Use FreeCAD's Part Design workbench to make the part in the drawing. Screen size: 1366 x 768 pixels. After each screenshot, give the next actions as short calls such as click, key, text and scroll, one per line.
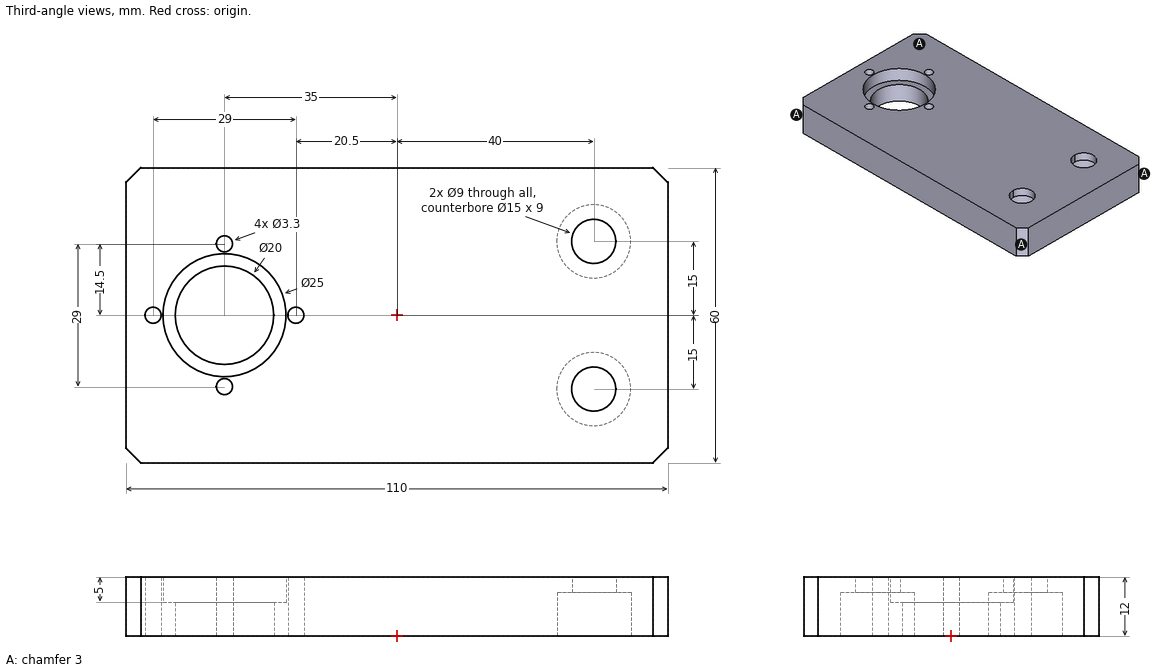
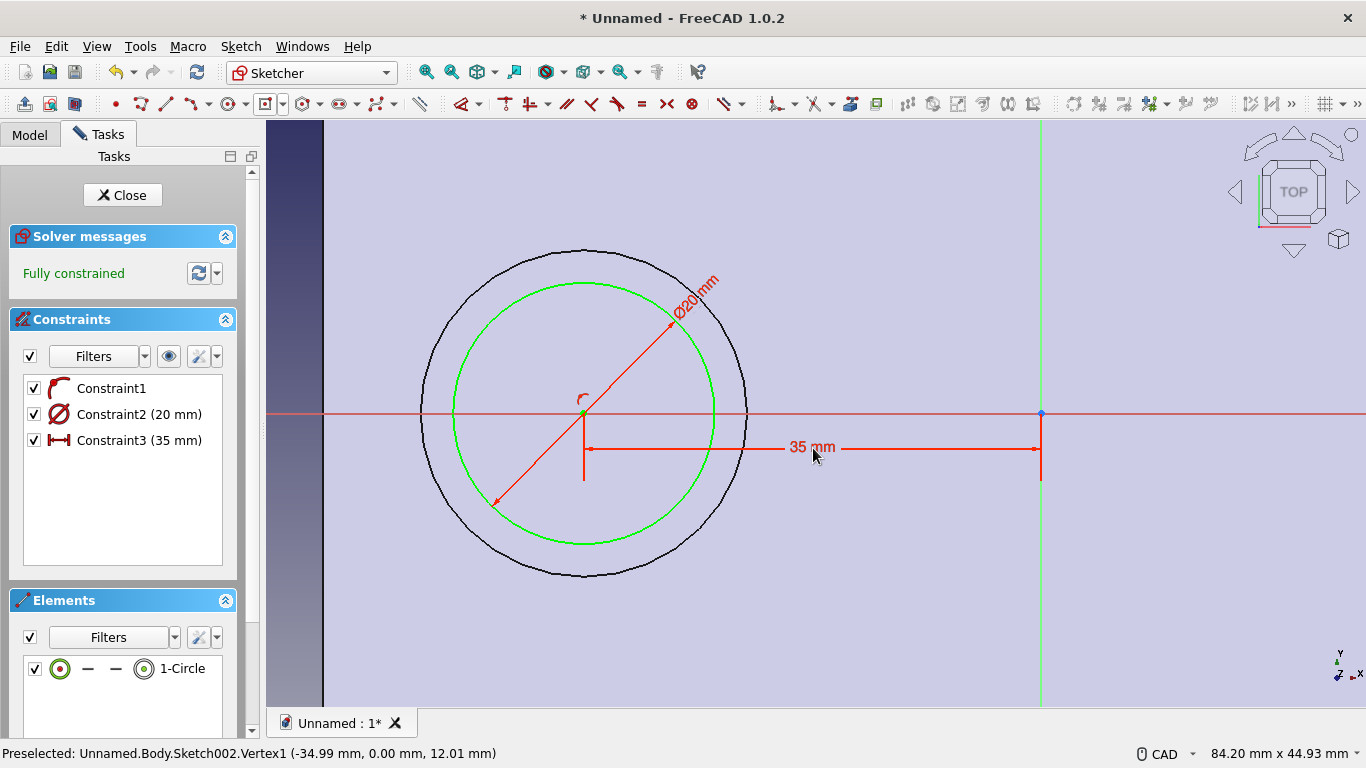
click(123, 195)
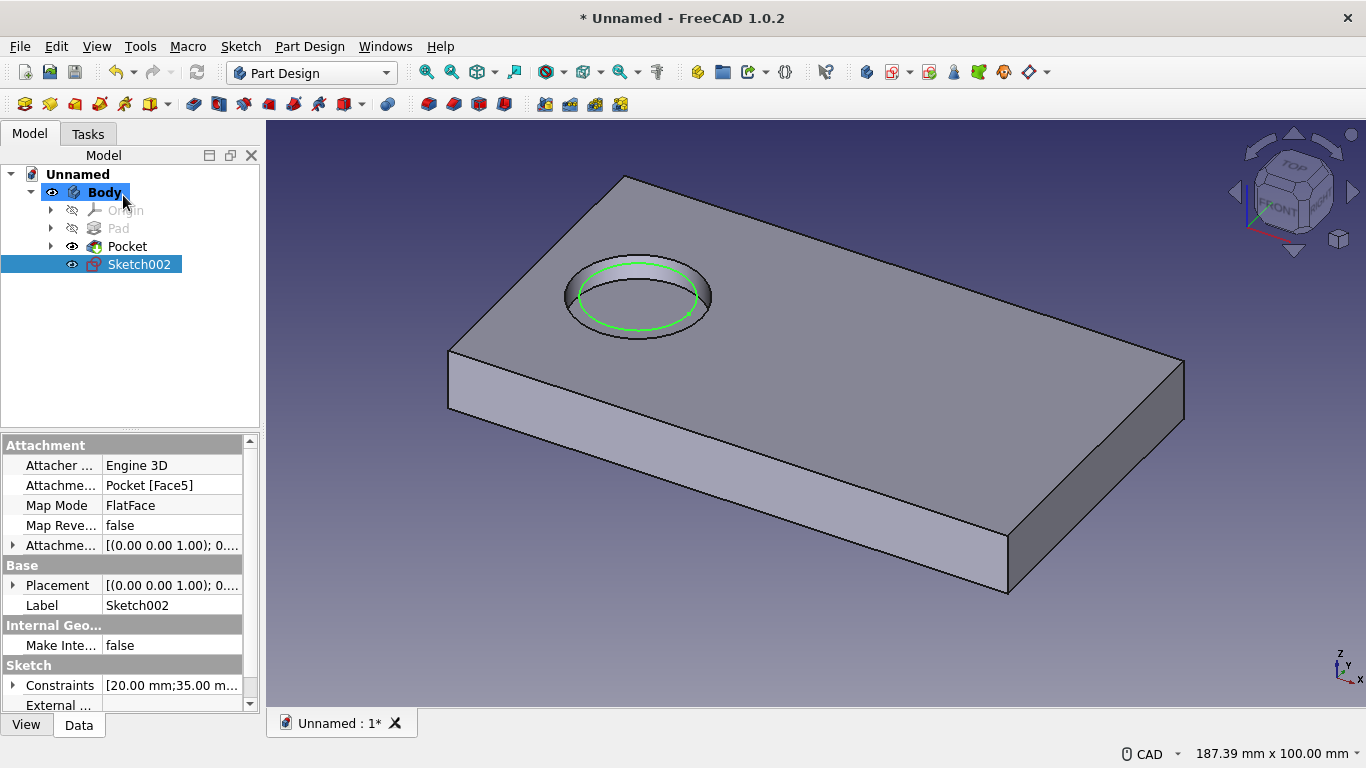
click(194, 104)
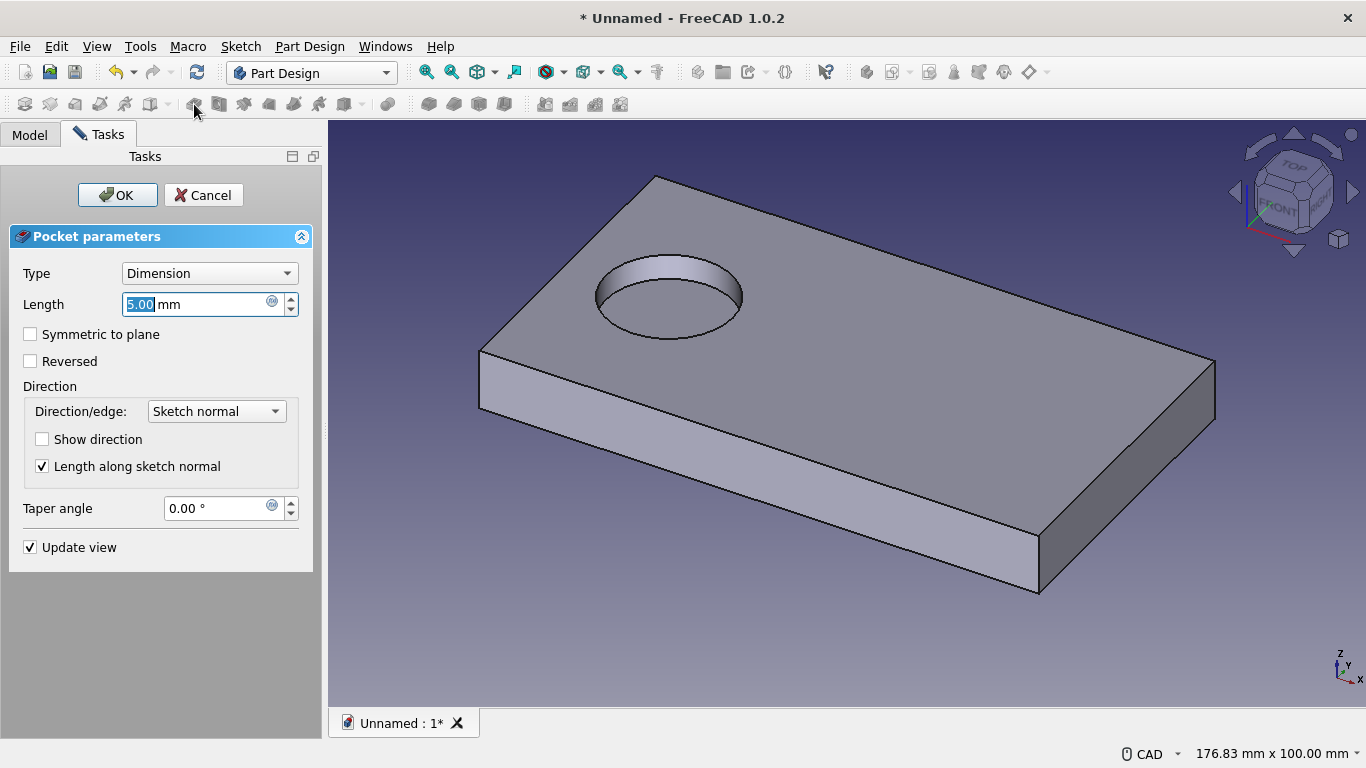
click(210, 274)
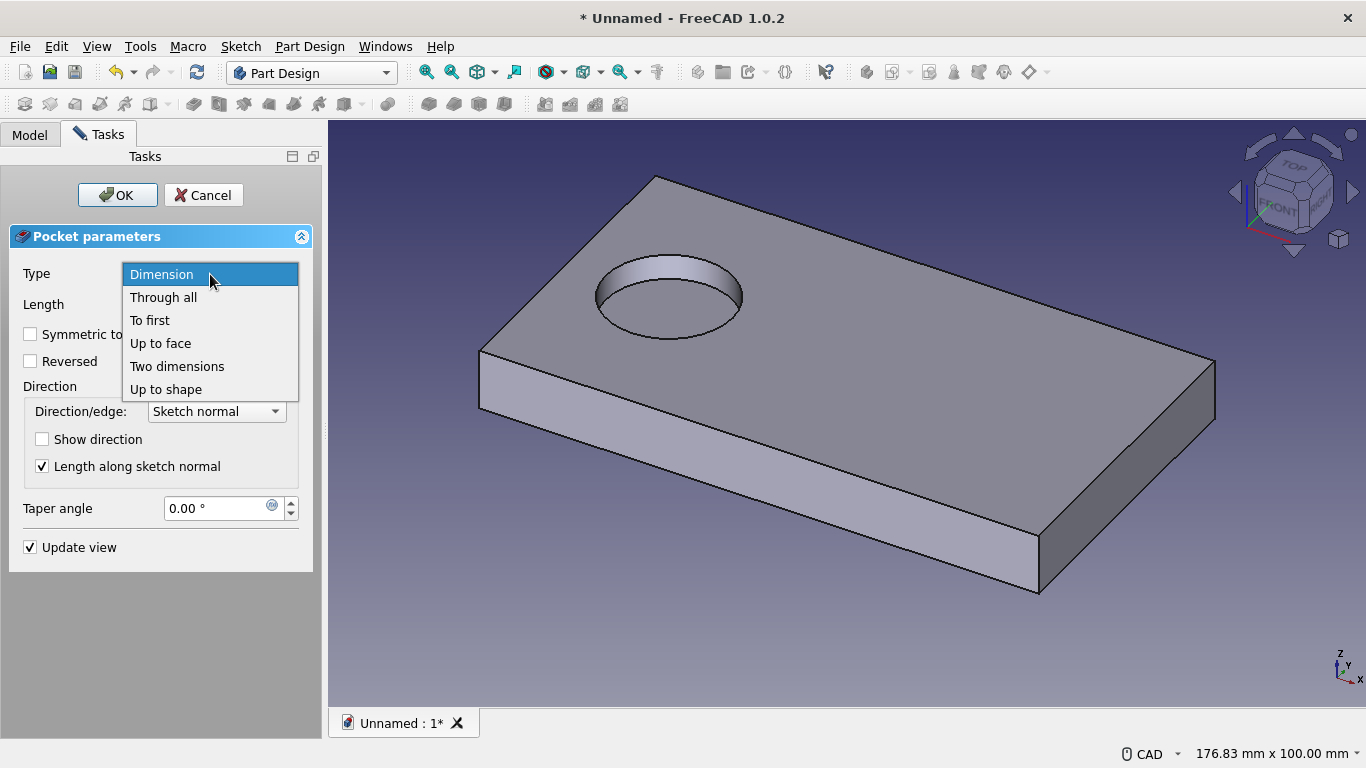
click(208, 298)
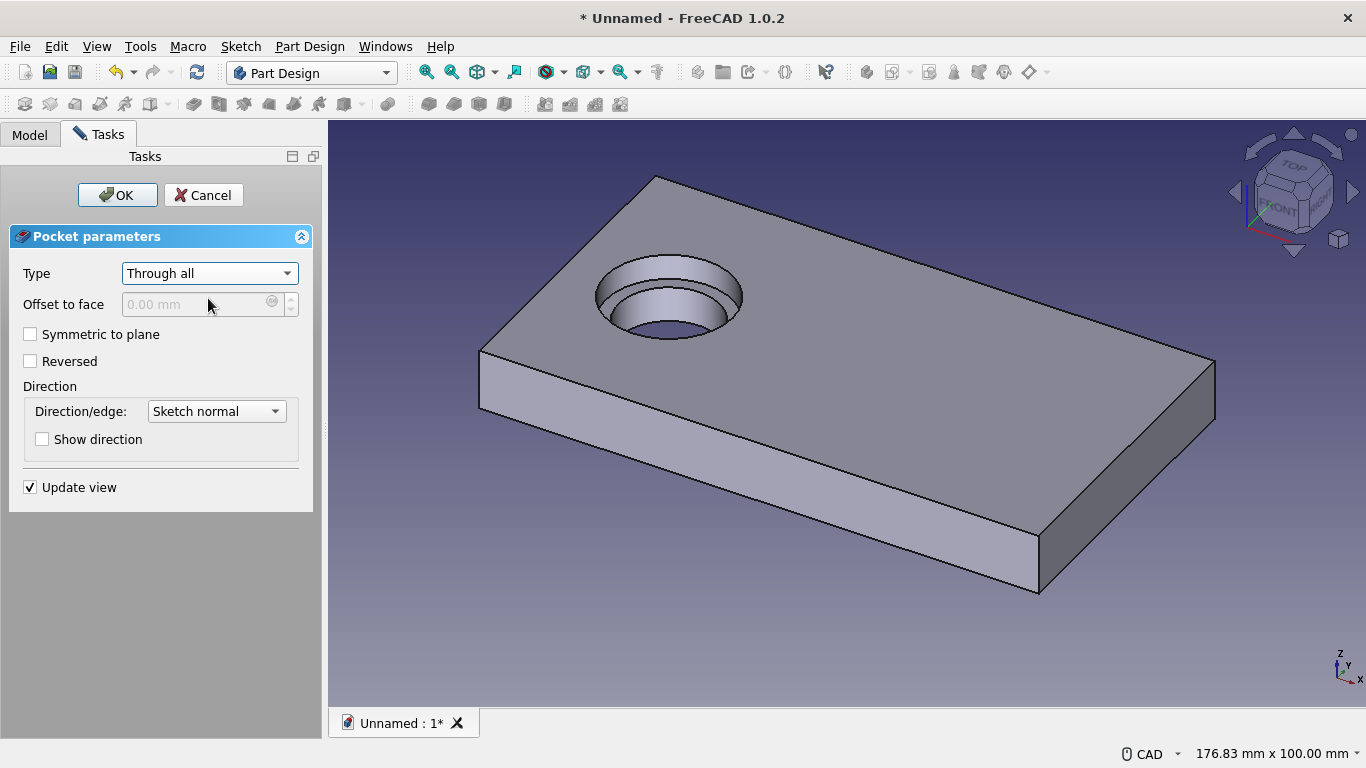
click(118, 195)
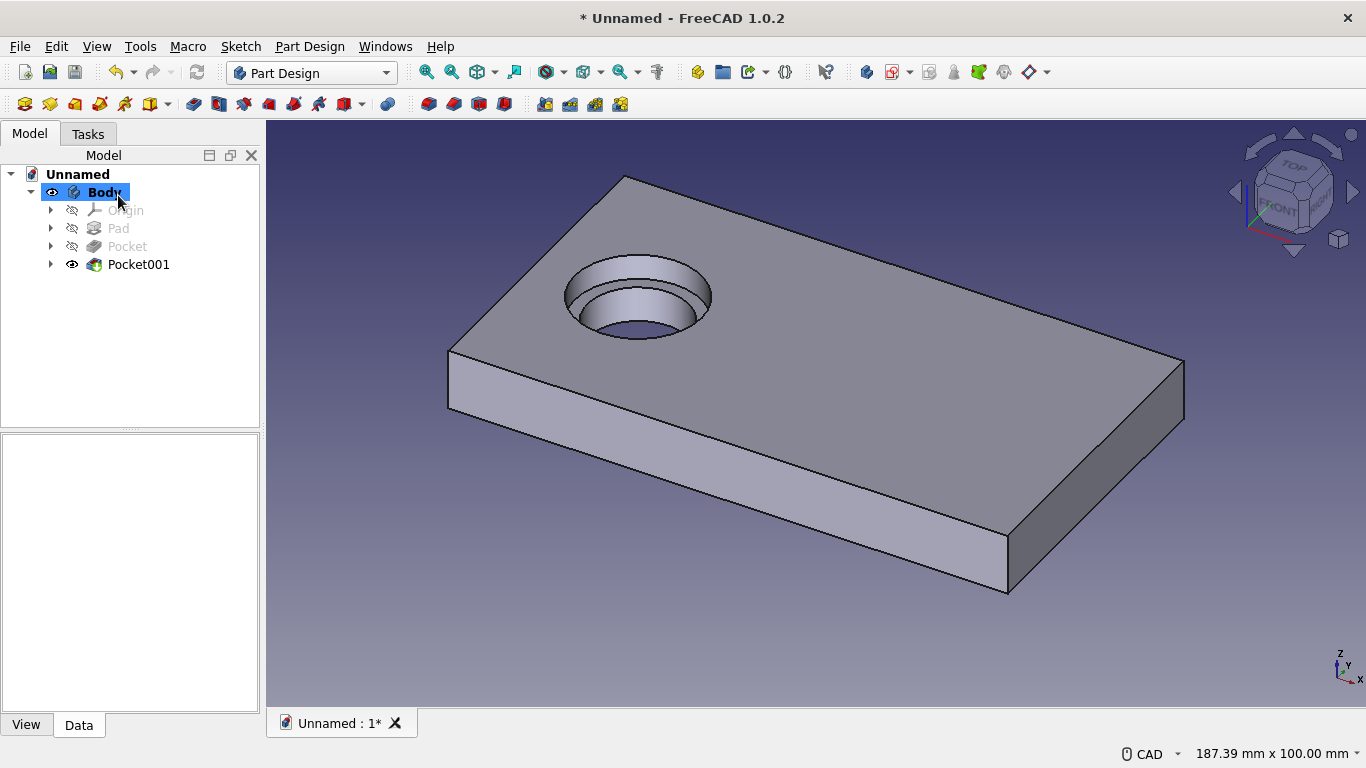
click(1008, 564)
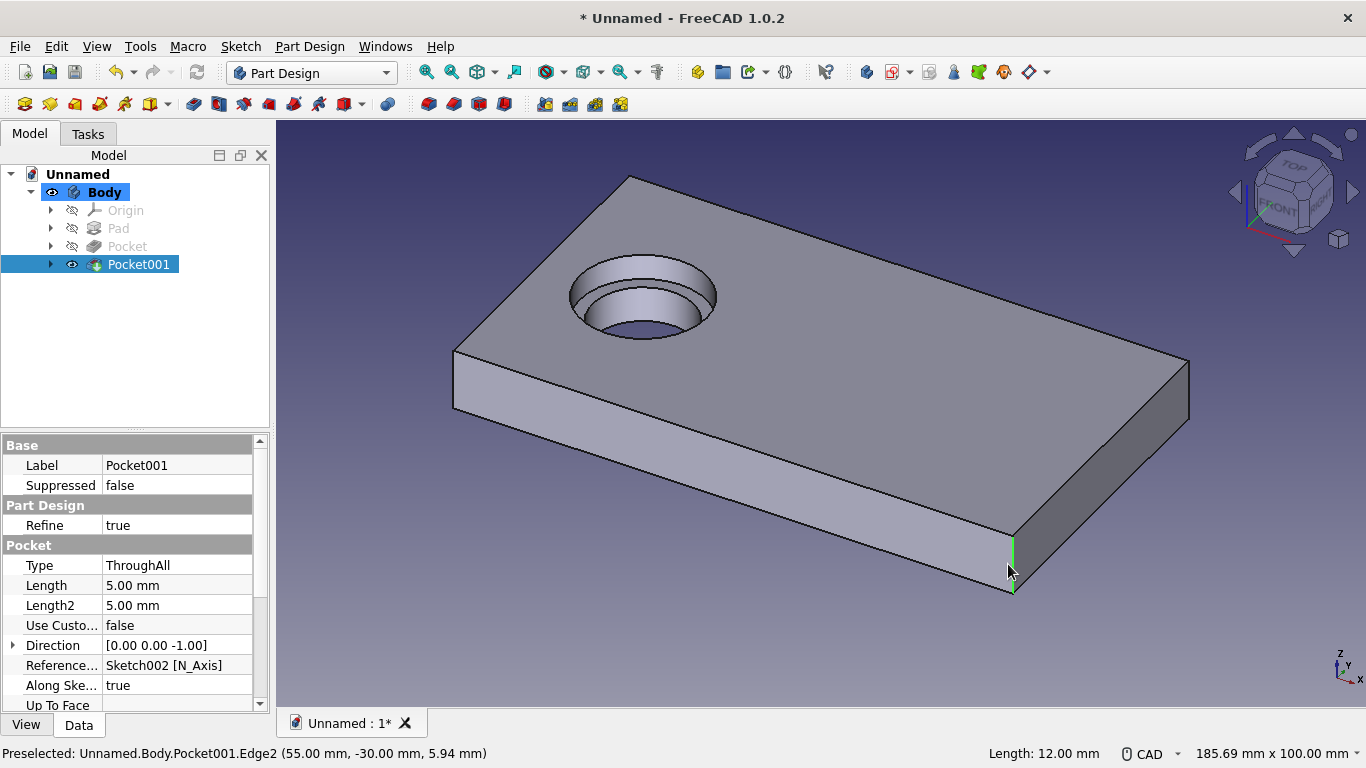
key(0)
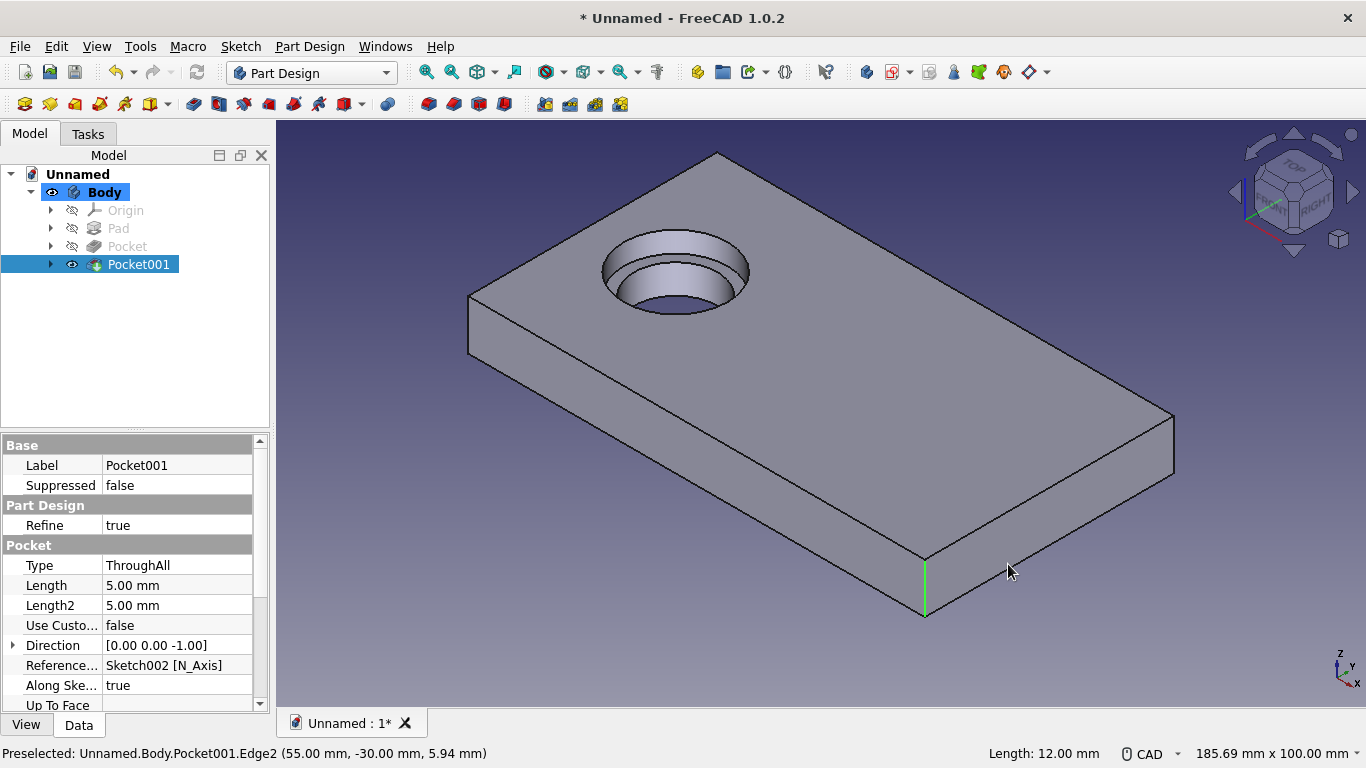
key(2)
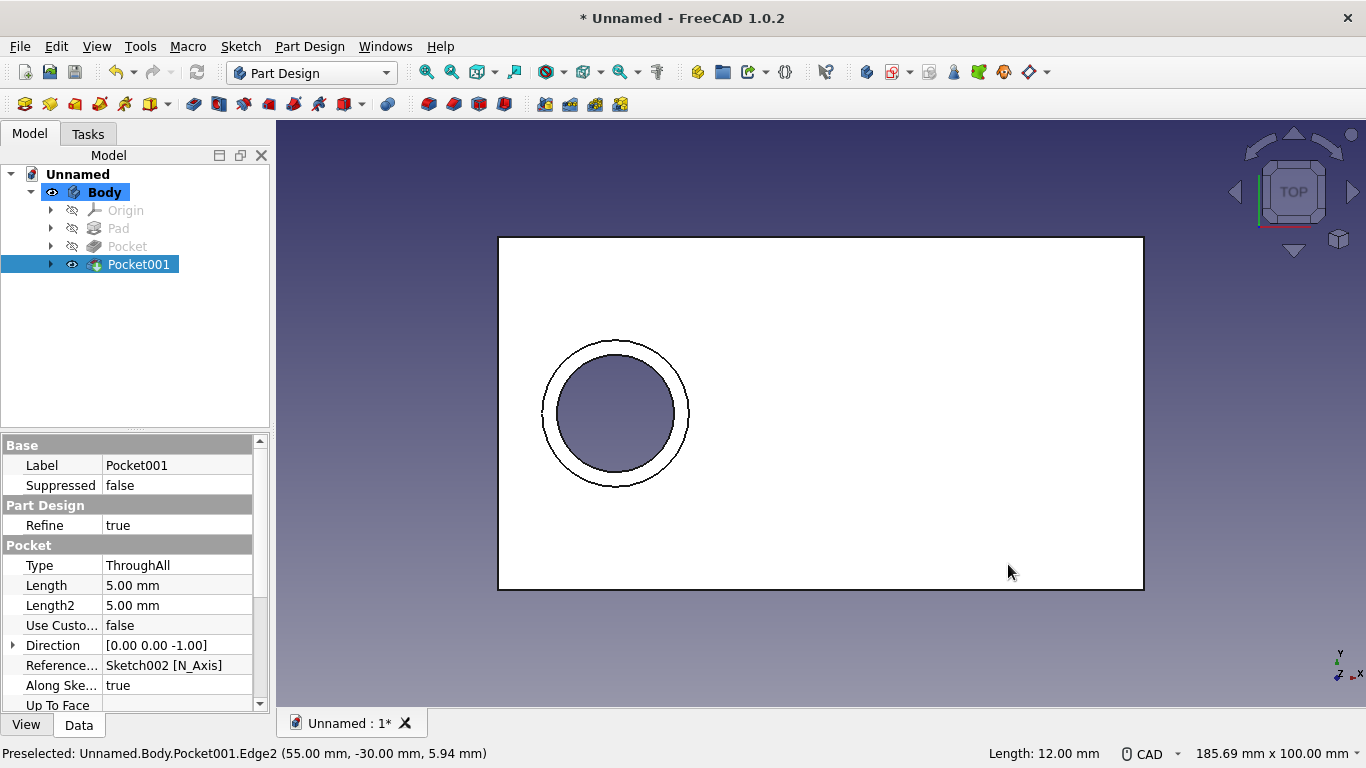
key(1)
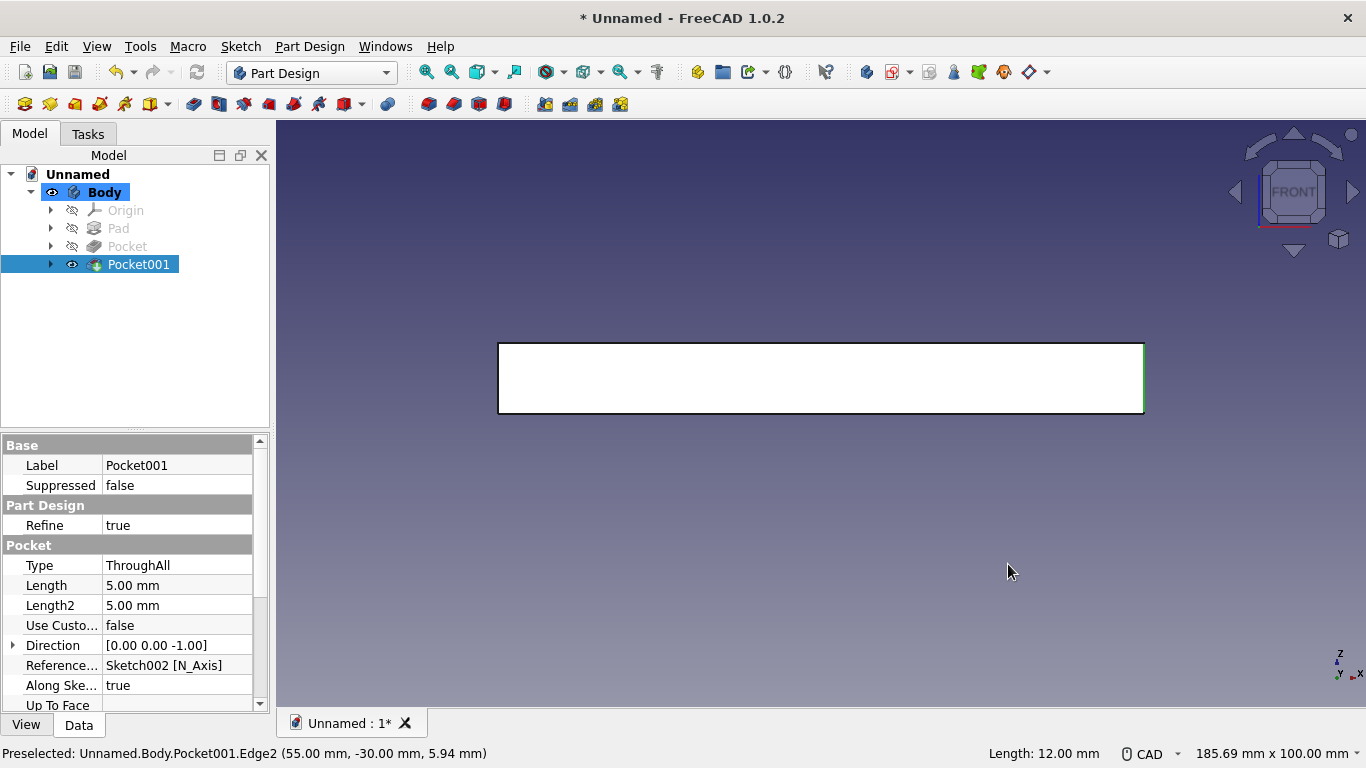
click(498, 377, ctrl)